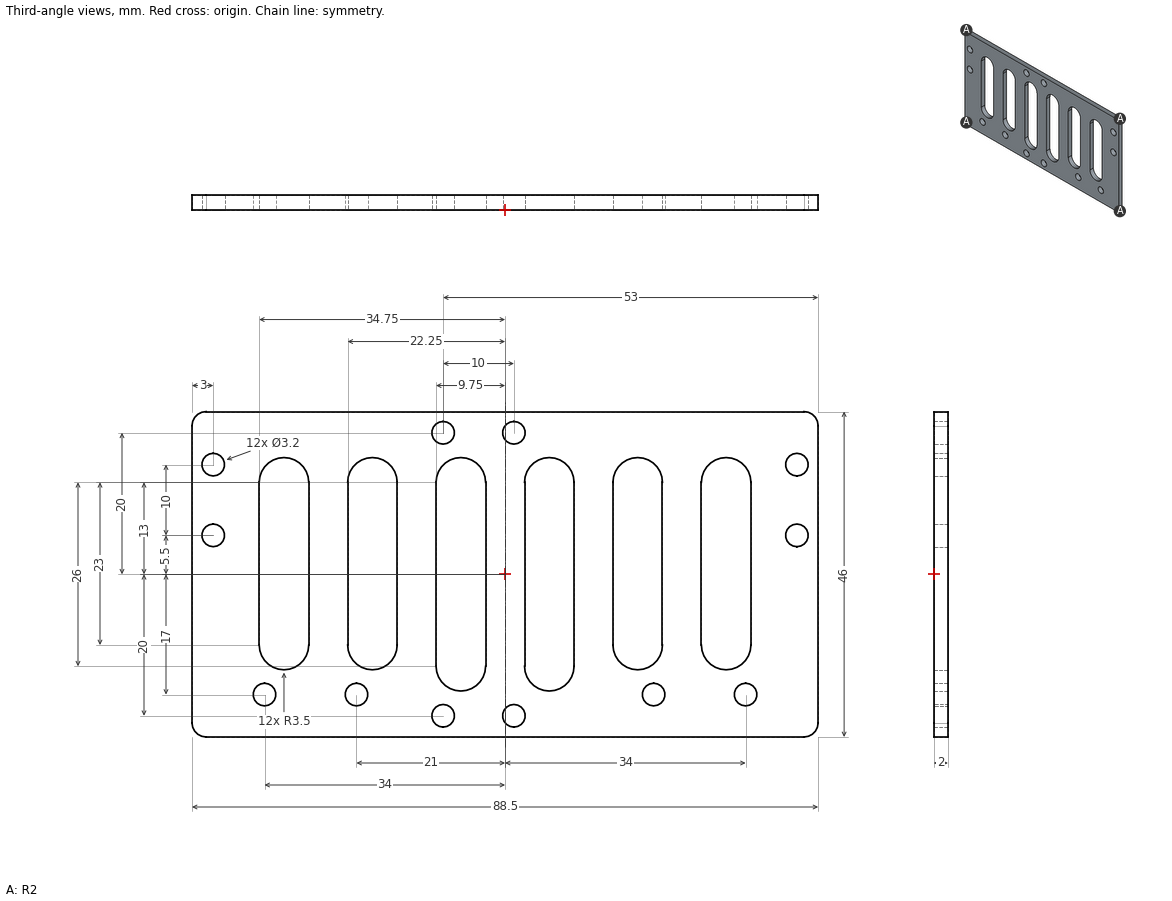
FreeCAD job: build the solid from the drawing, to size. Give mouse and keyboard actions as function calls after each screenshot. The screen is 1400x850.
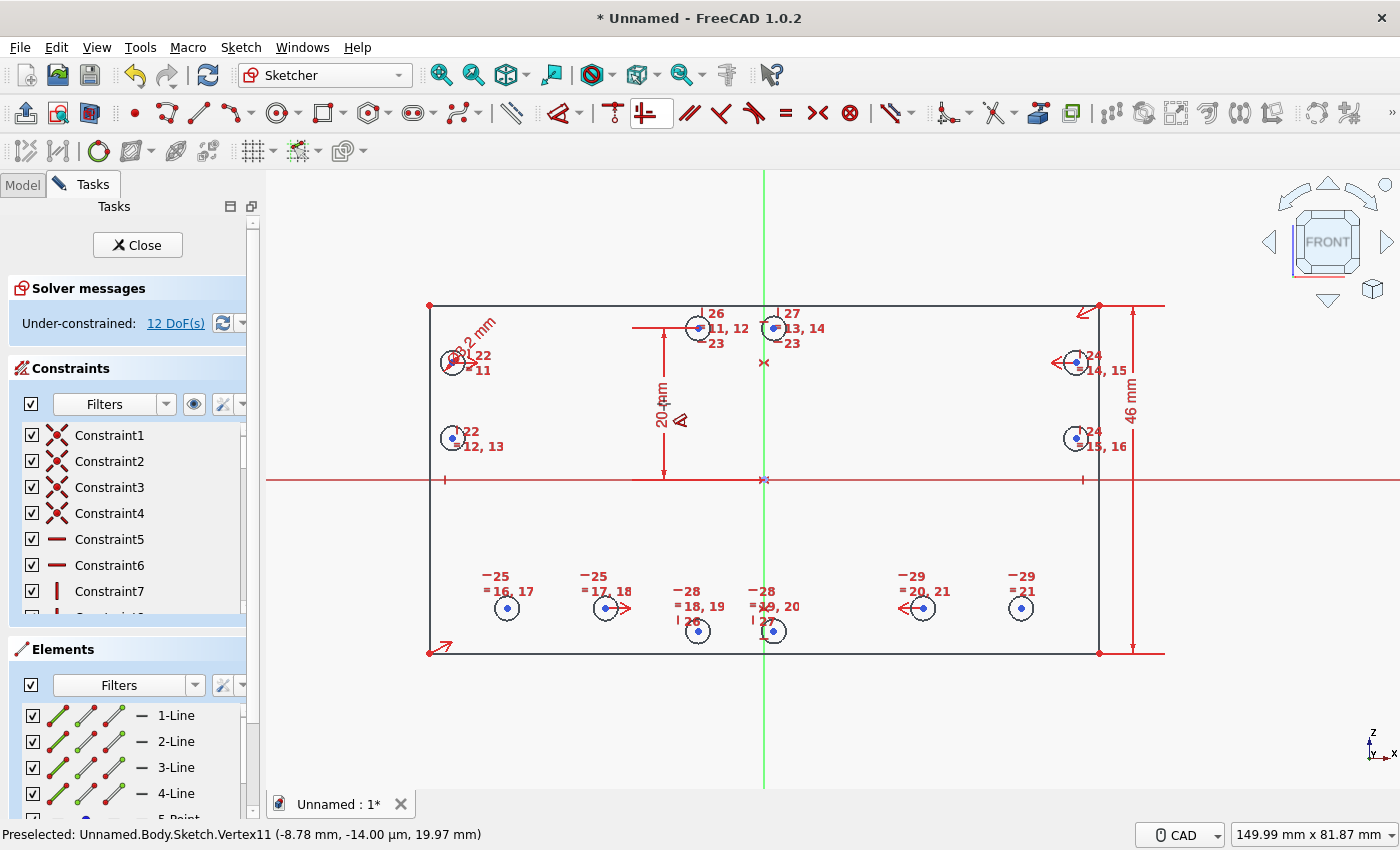
click(507, 608)
click(636, 446)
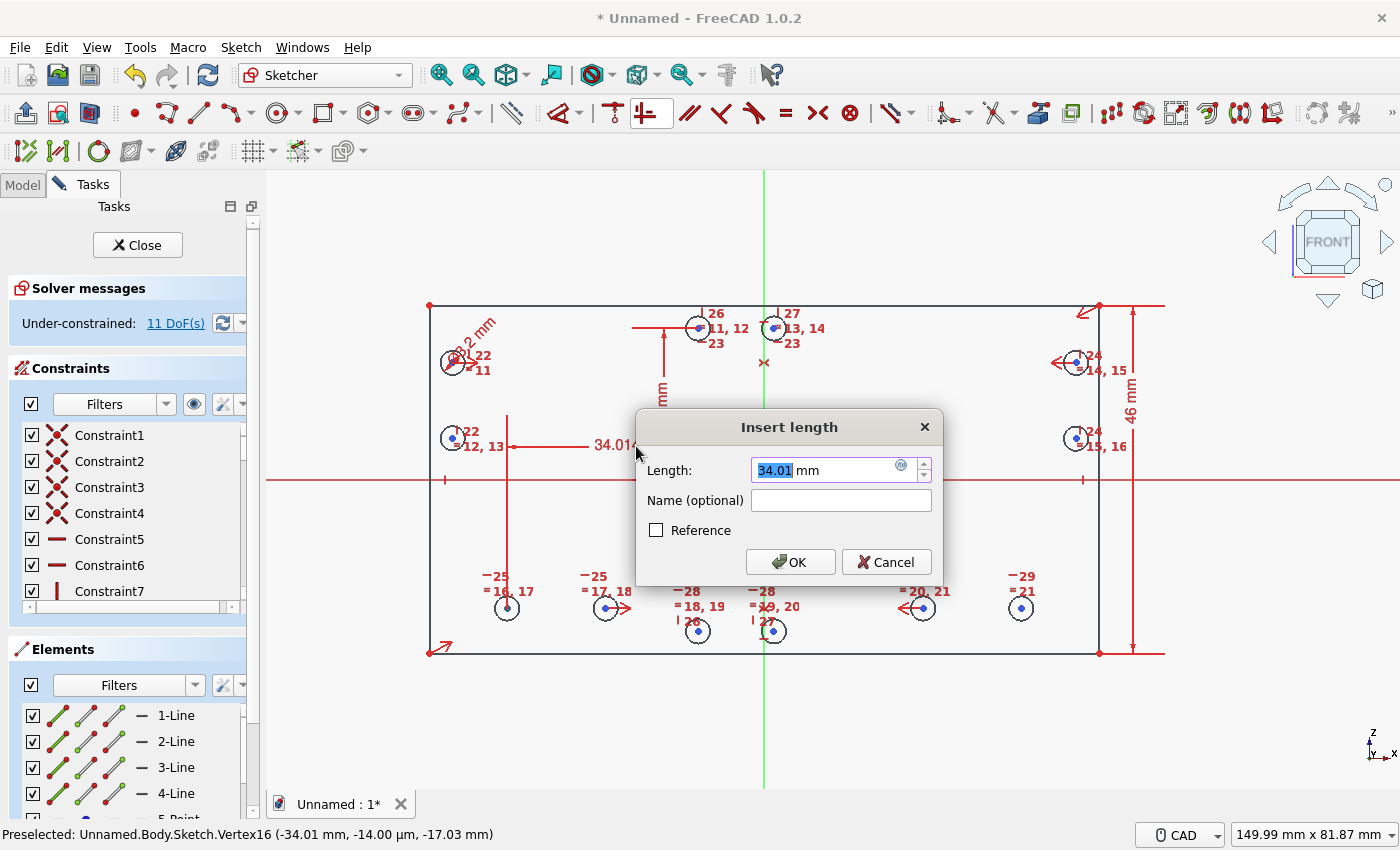
text(34)
key(Return)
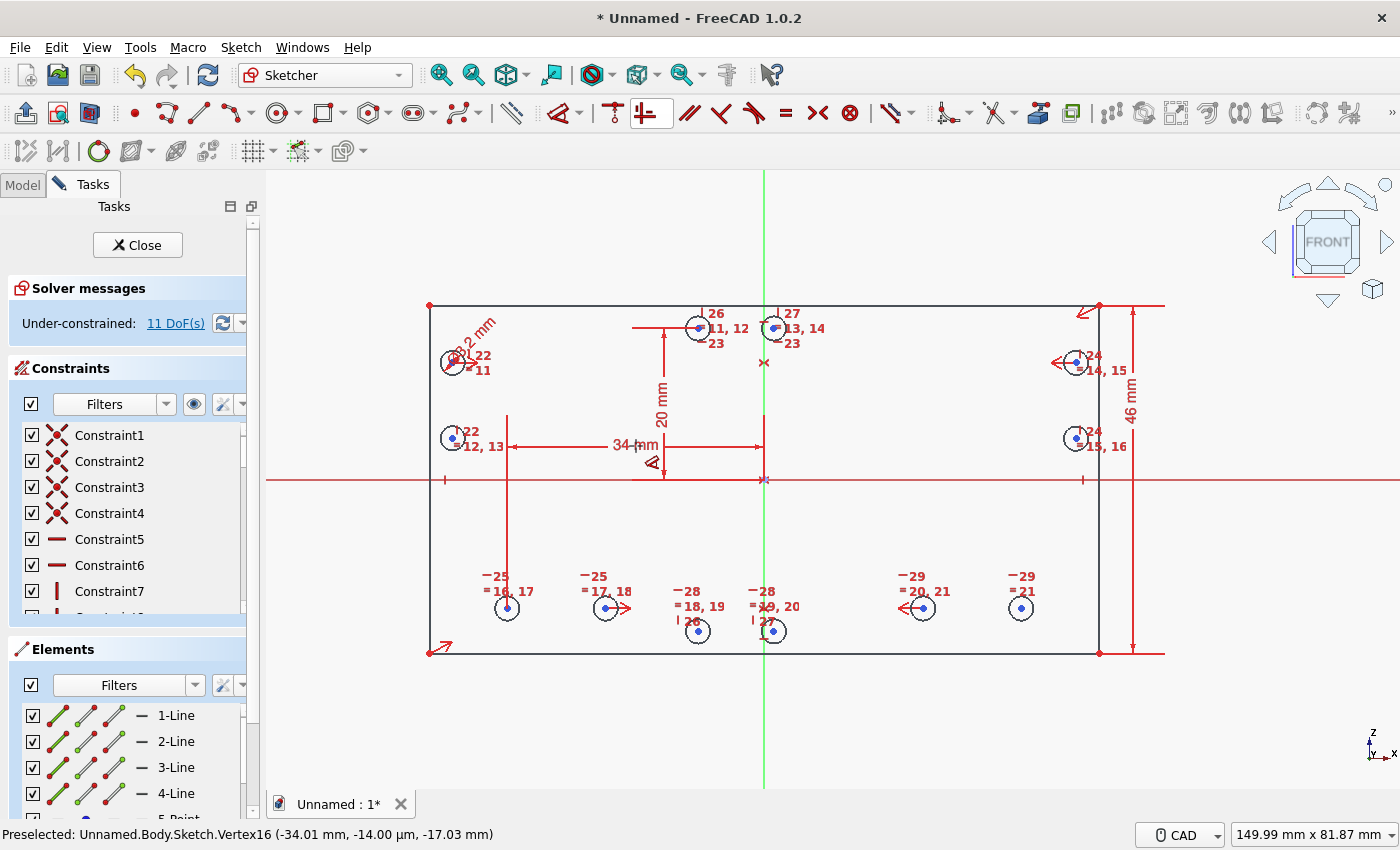
click(507, 608)
click(473, 544)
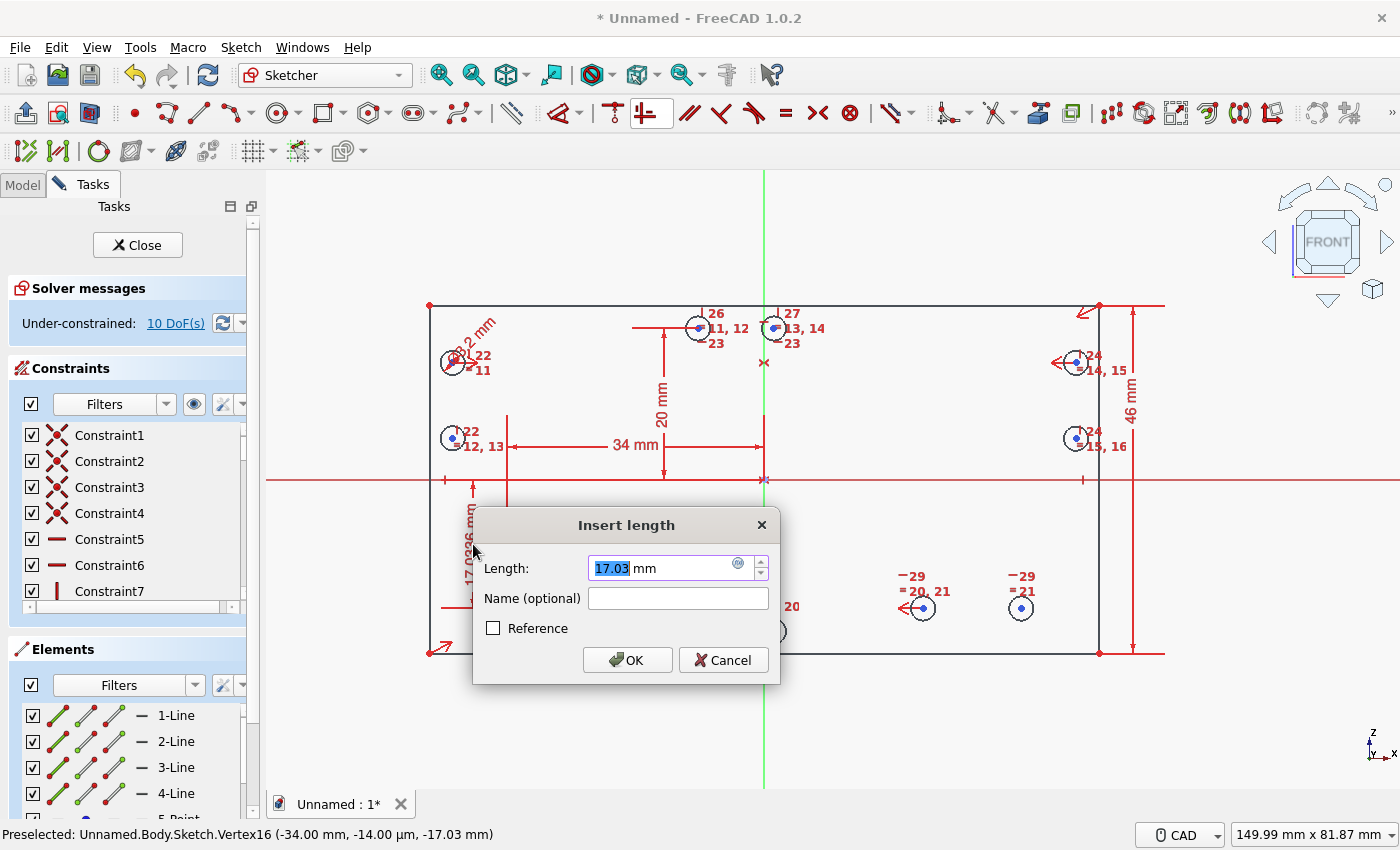
text(17)
key(Return)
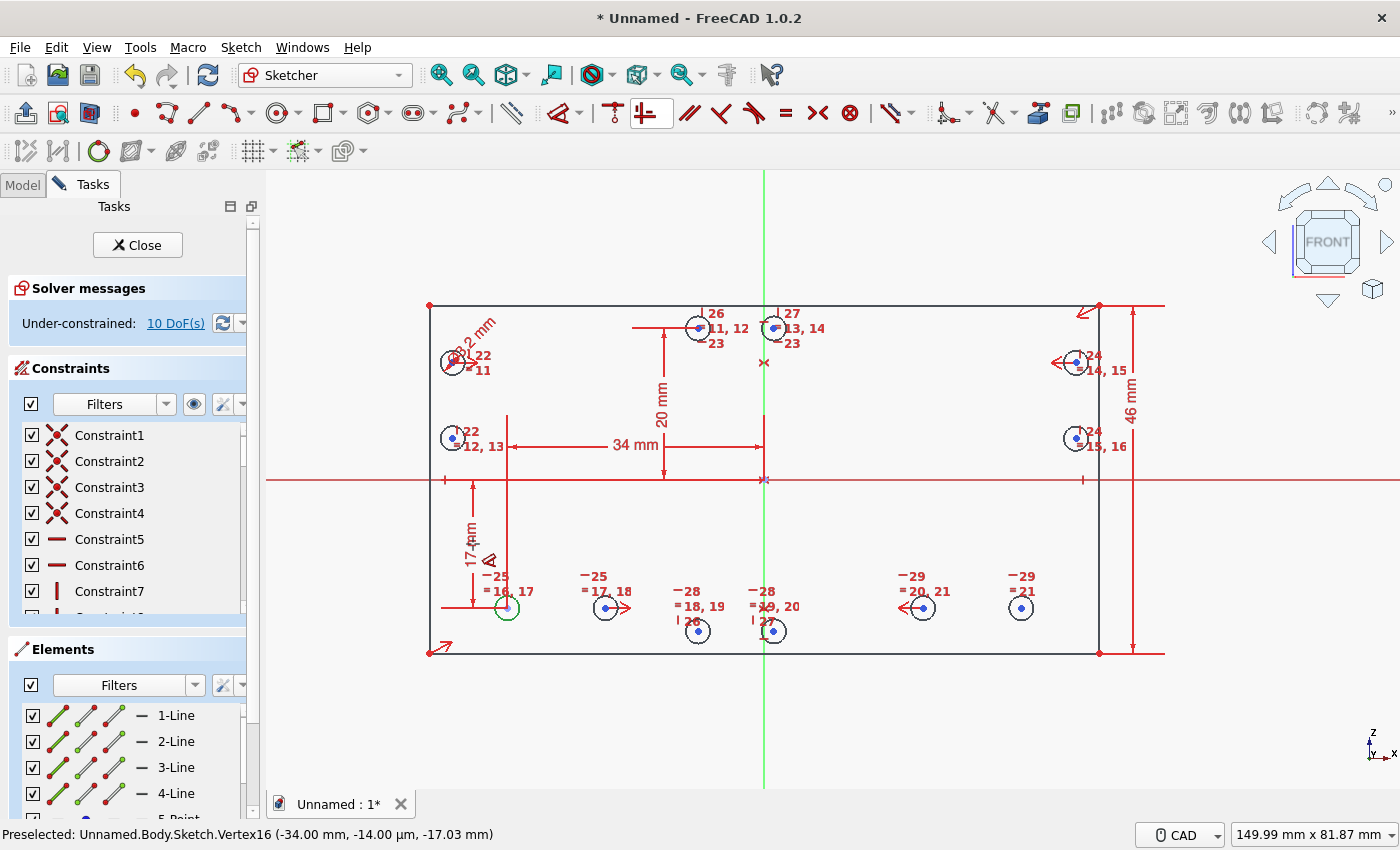
click(606, 608)
click(722, 446)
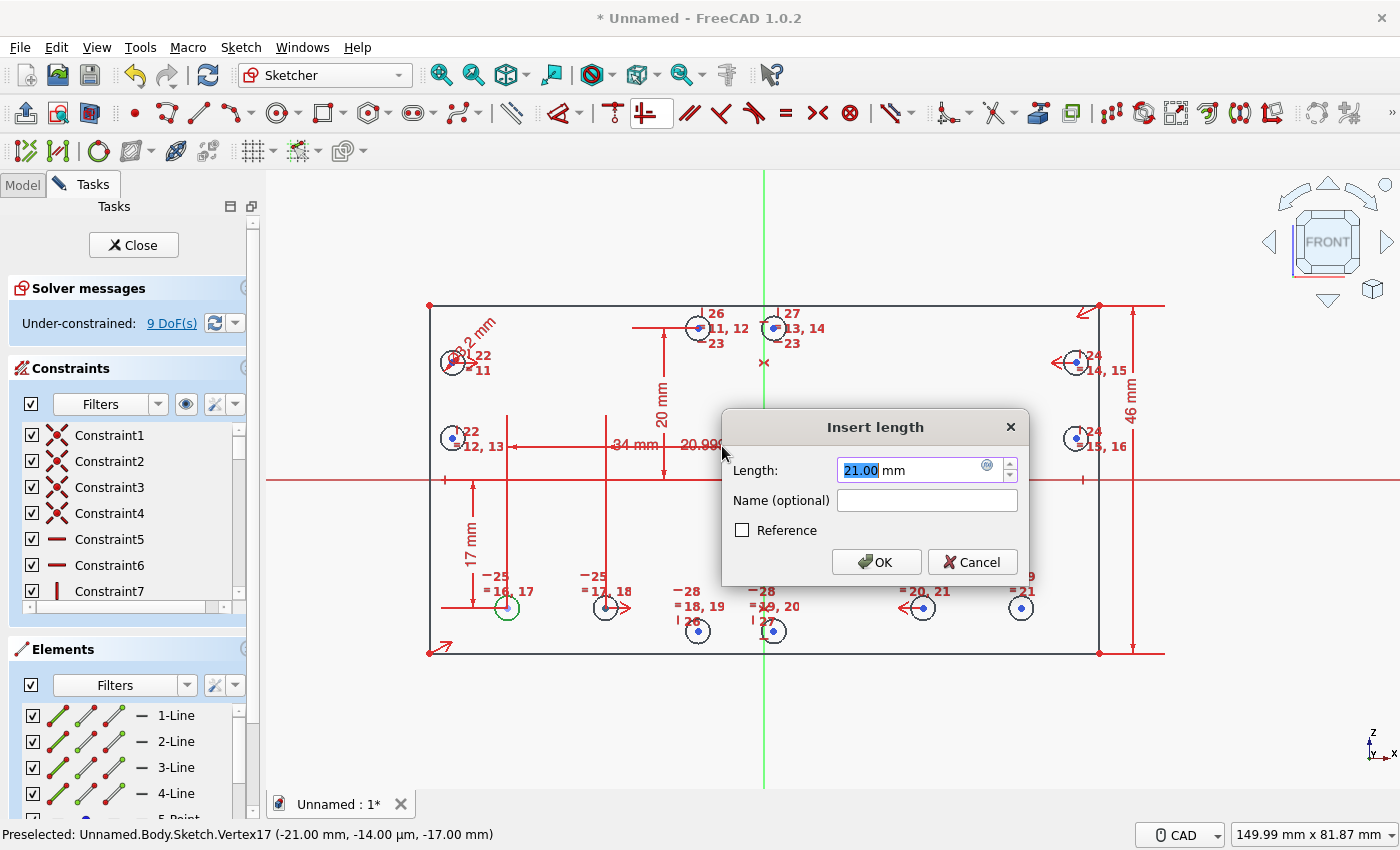
text(21)
key(Return)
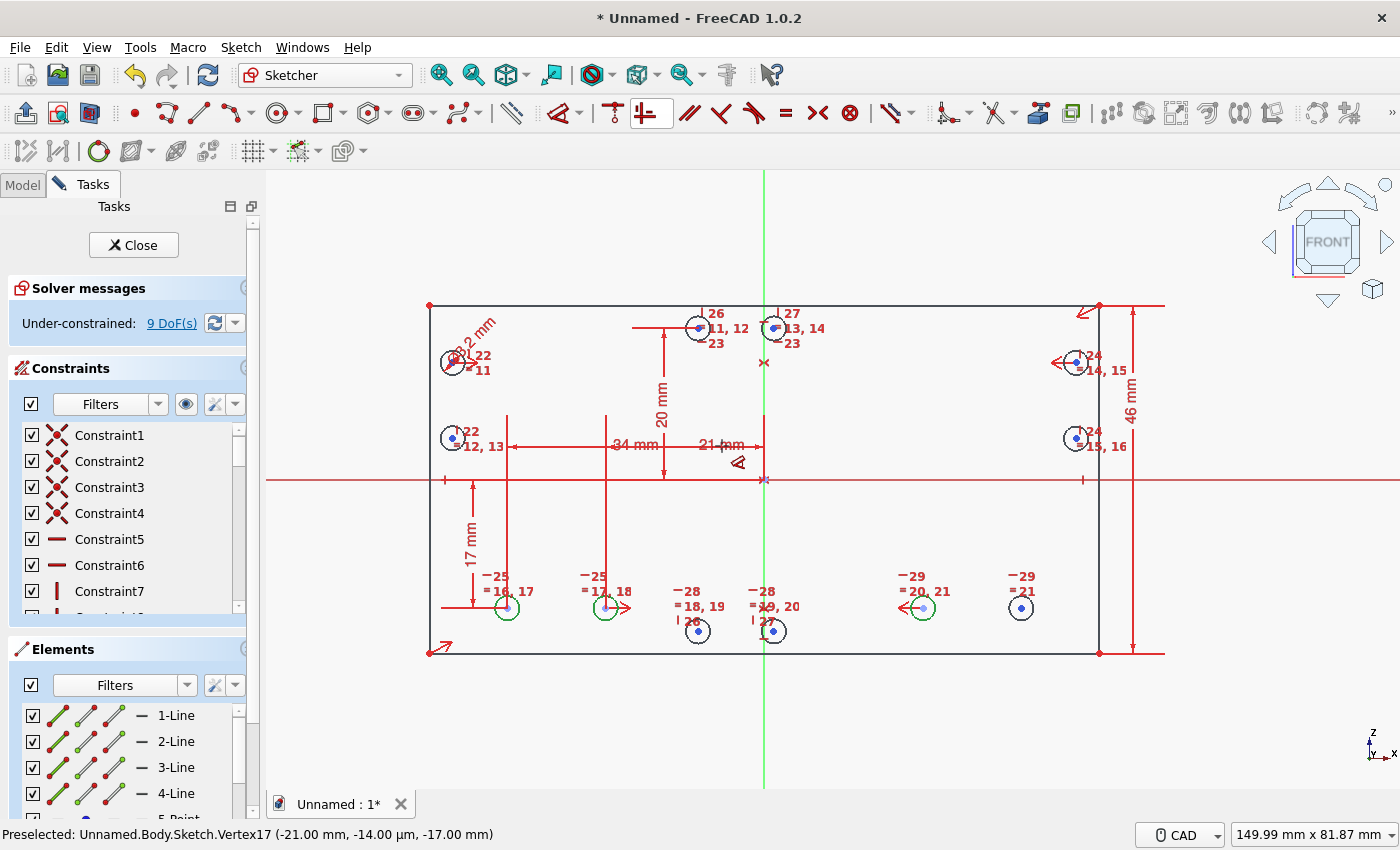
click(698, 631)
click(664, 556)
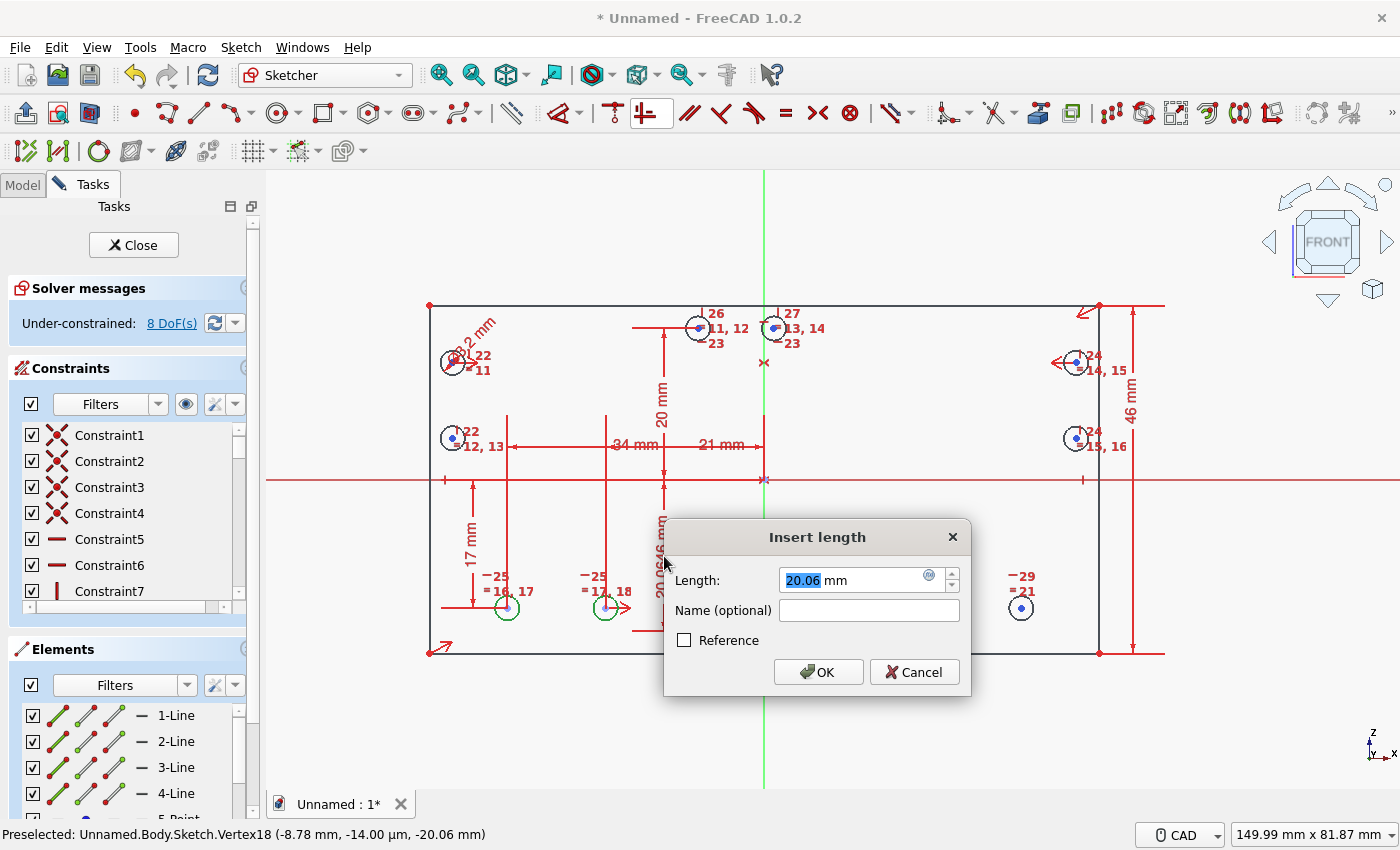
text(20)
key(Return)